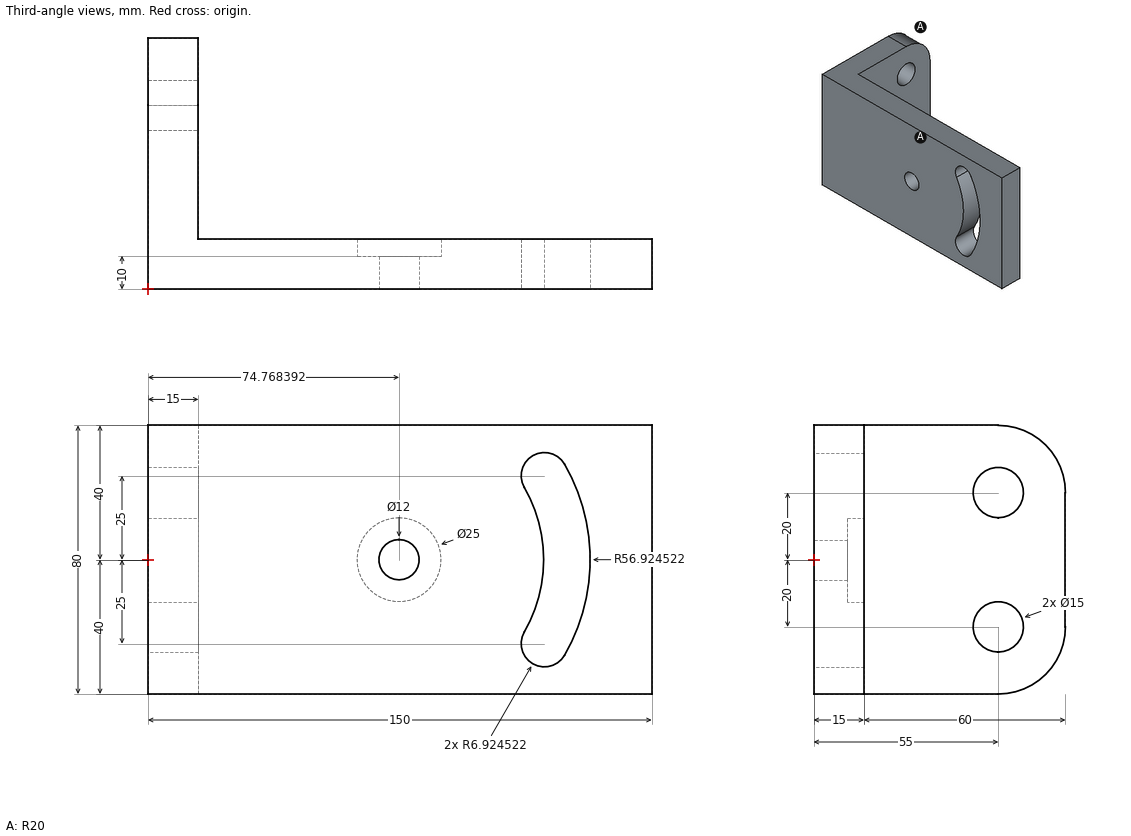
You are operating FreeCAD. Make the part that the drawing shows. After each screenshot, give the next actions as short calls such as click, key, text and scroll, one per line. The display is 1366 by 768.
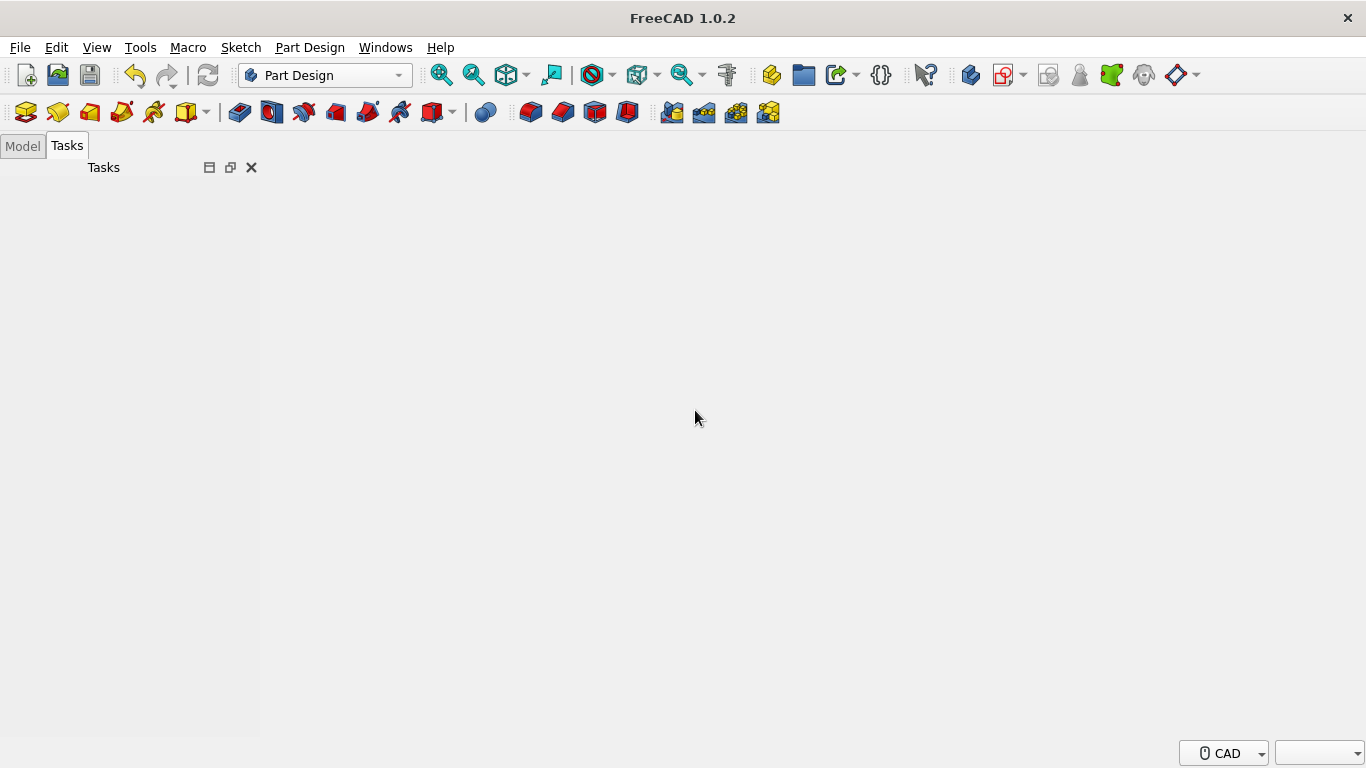
key(ctrl+n)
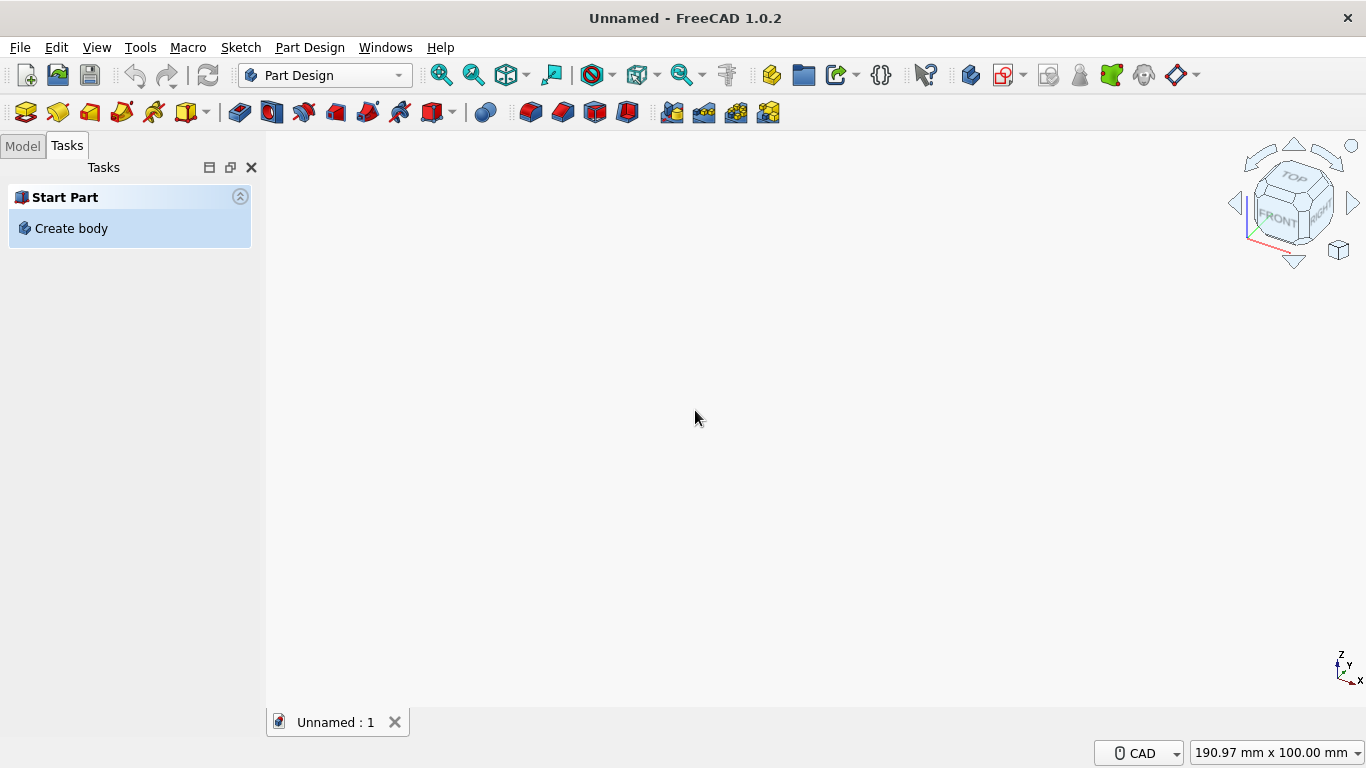
click(1004, 76)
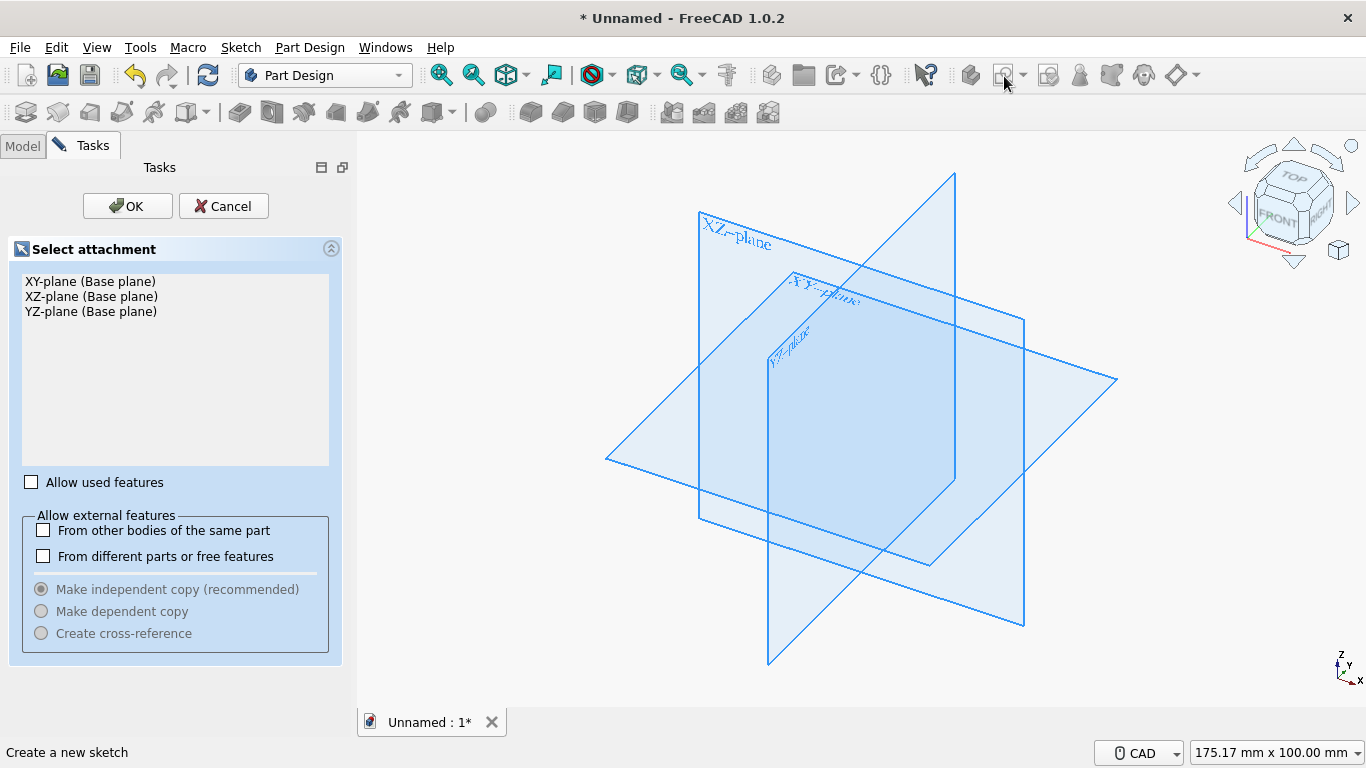
click(82, 296)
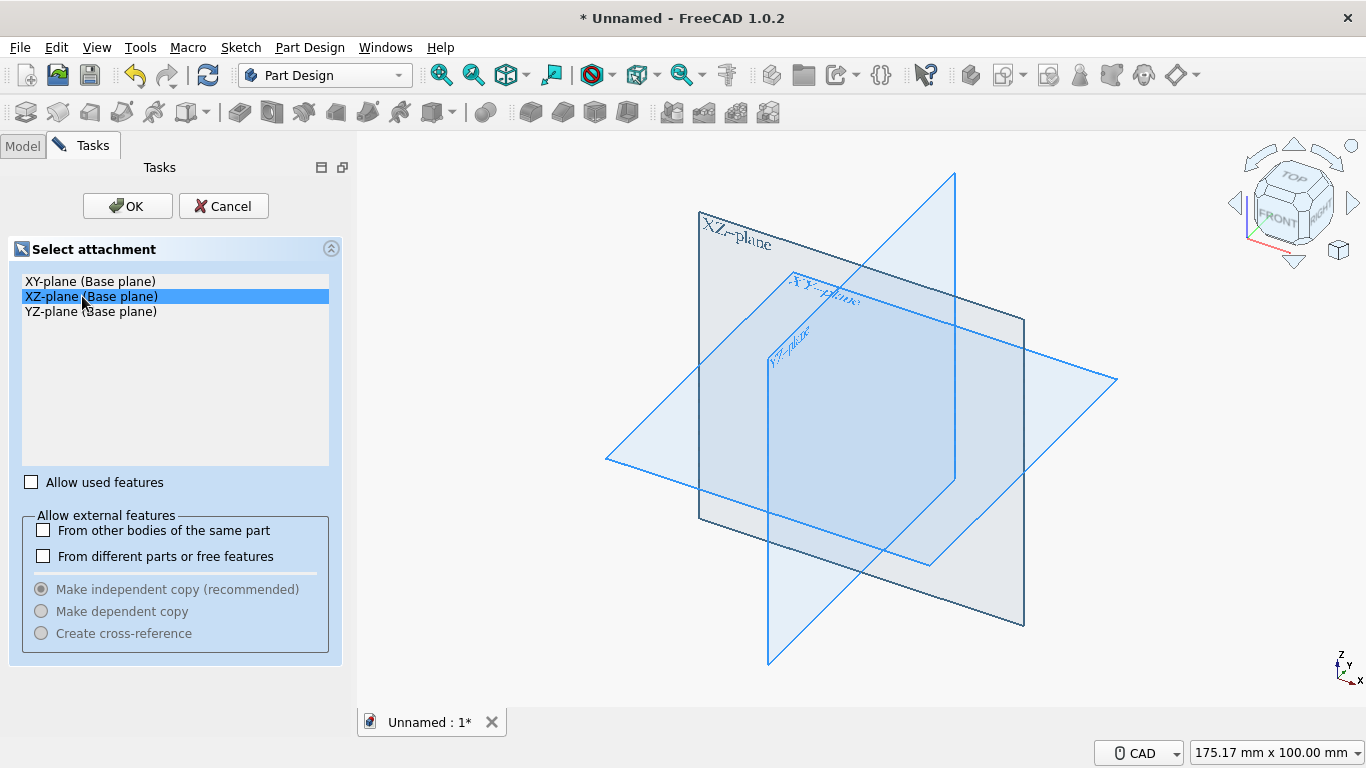
click(128, 206)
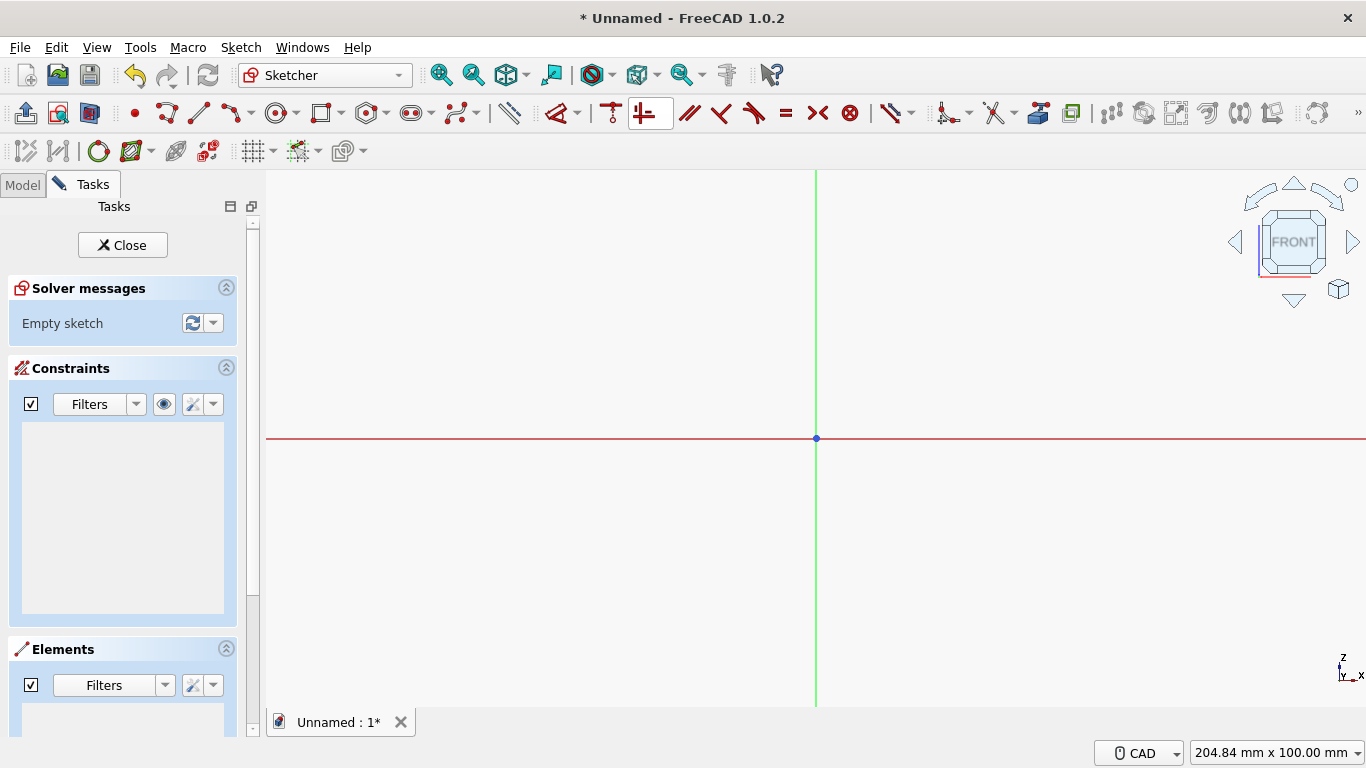
scroll(294, 438, down, 3)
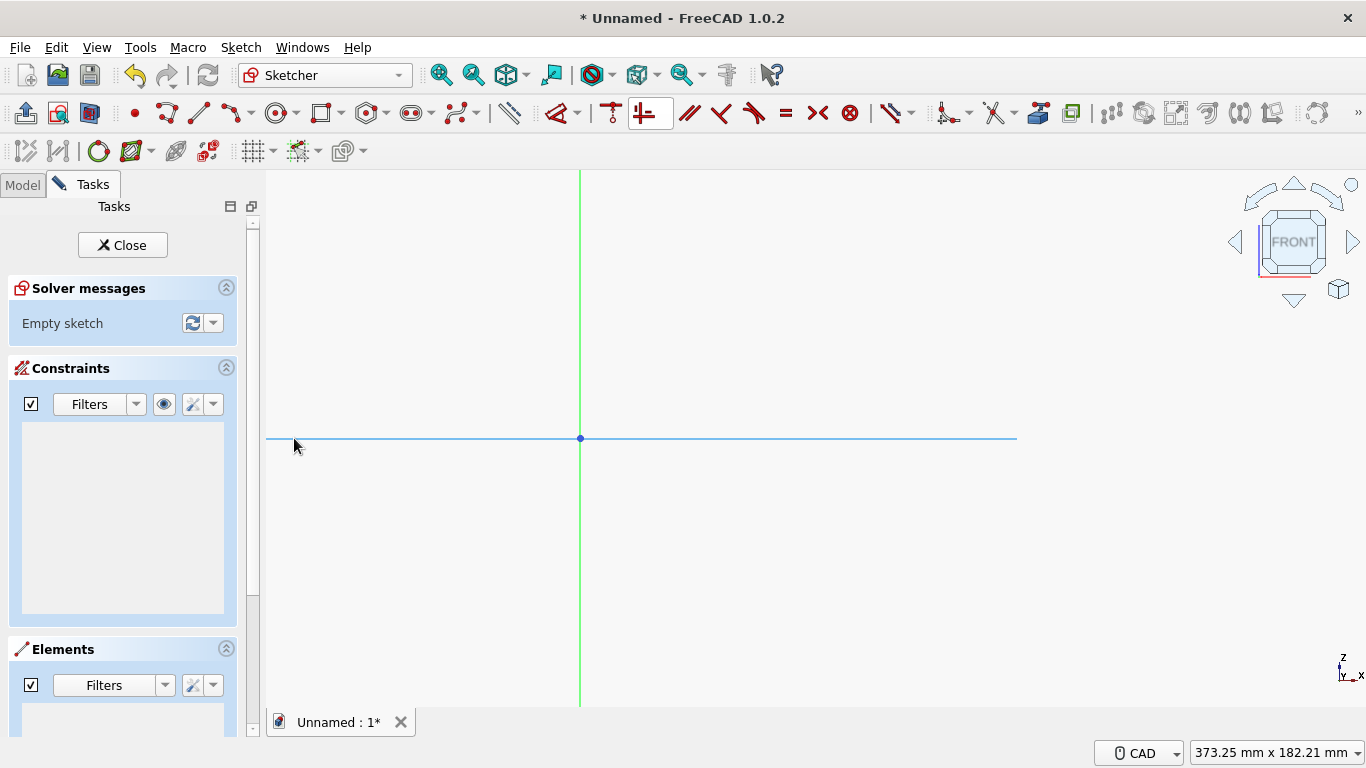
scroll(911, 439, up, 2)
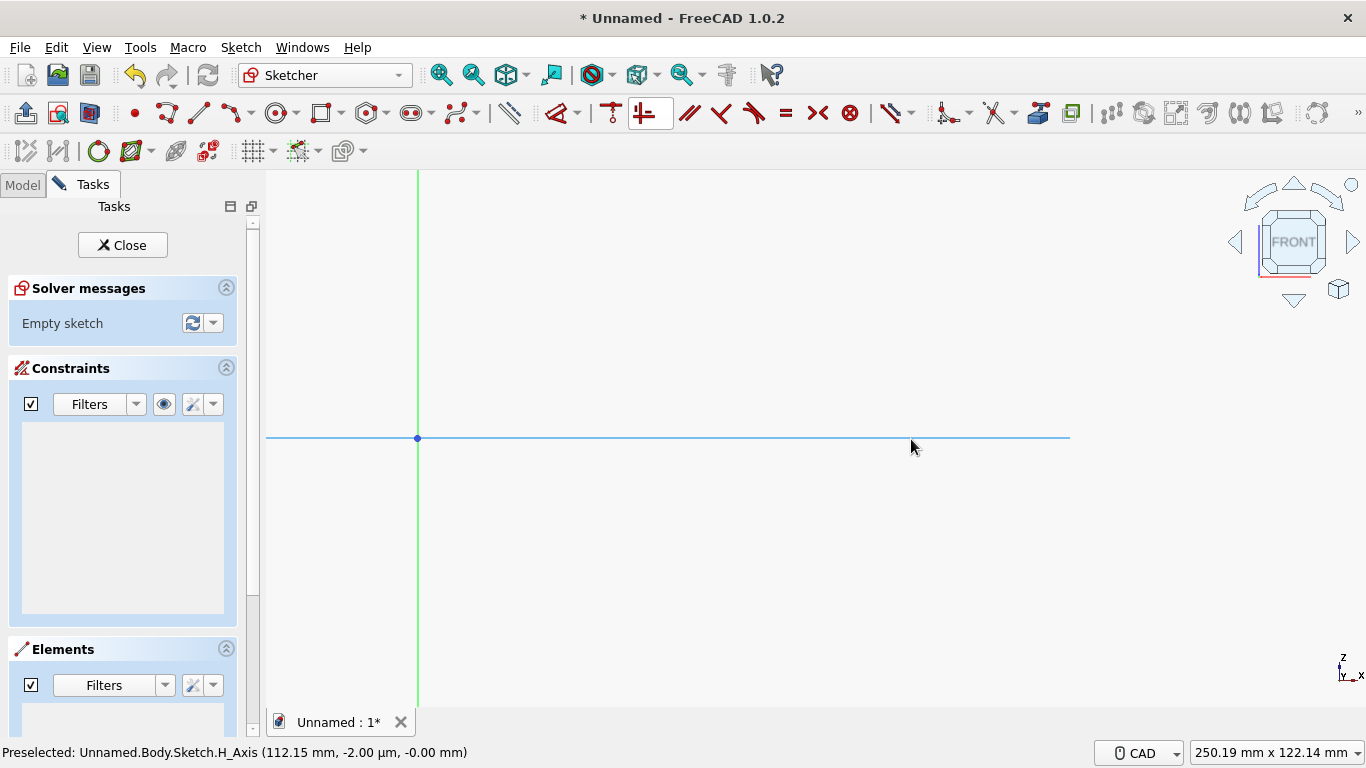
click(322, 114)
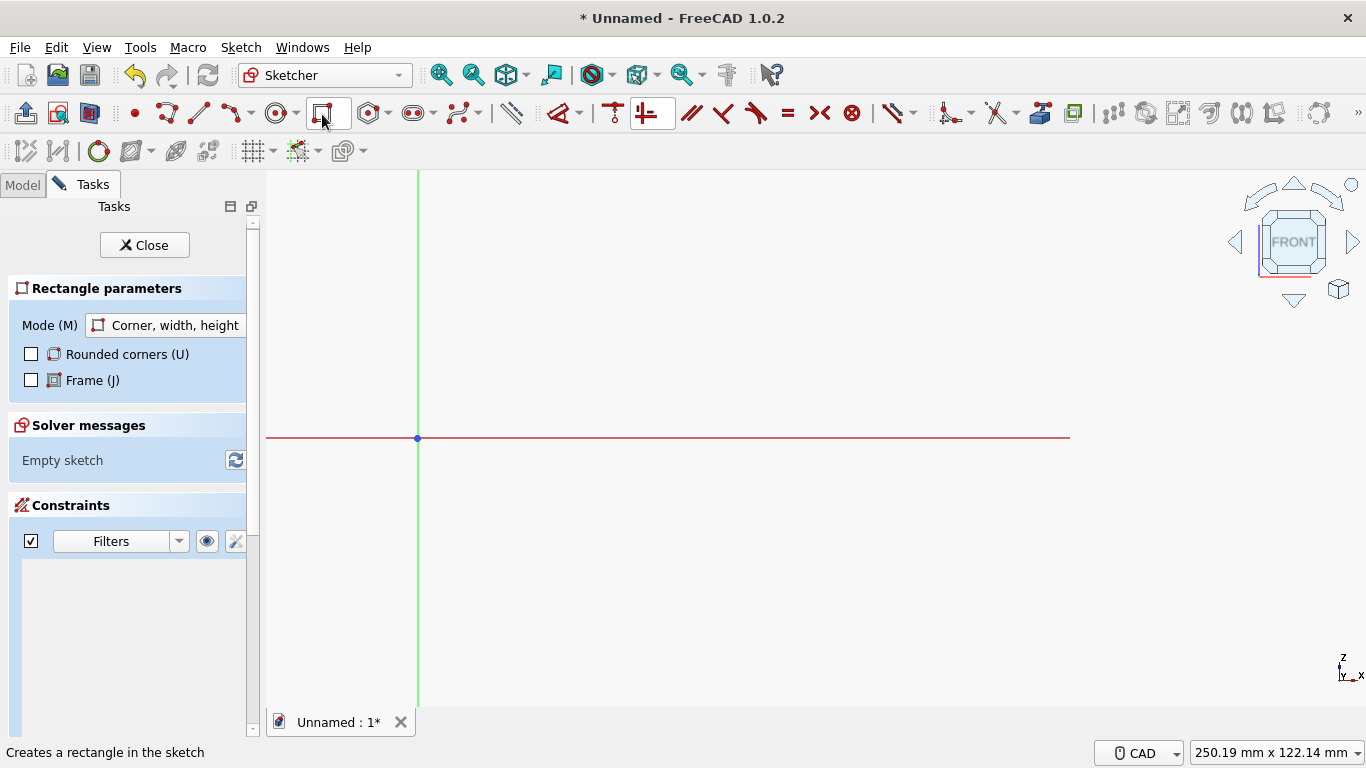
click(418, 262)
click(1077, 614)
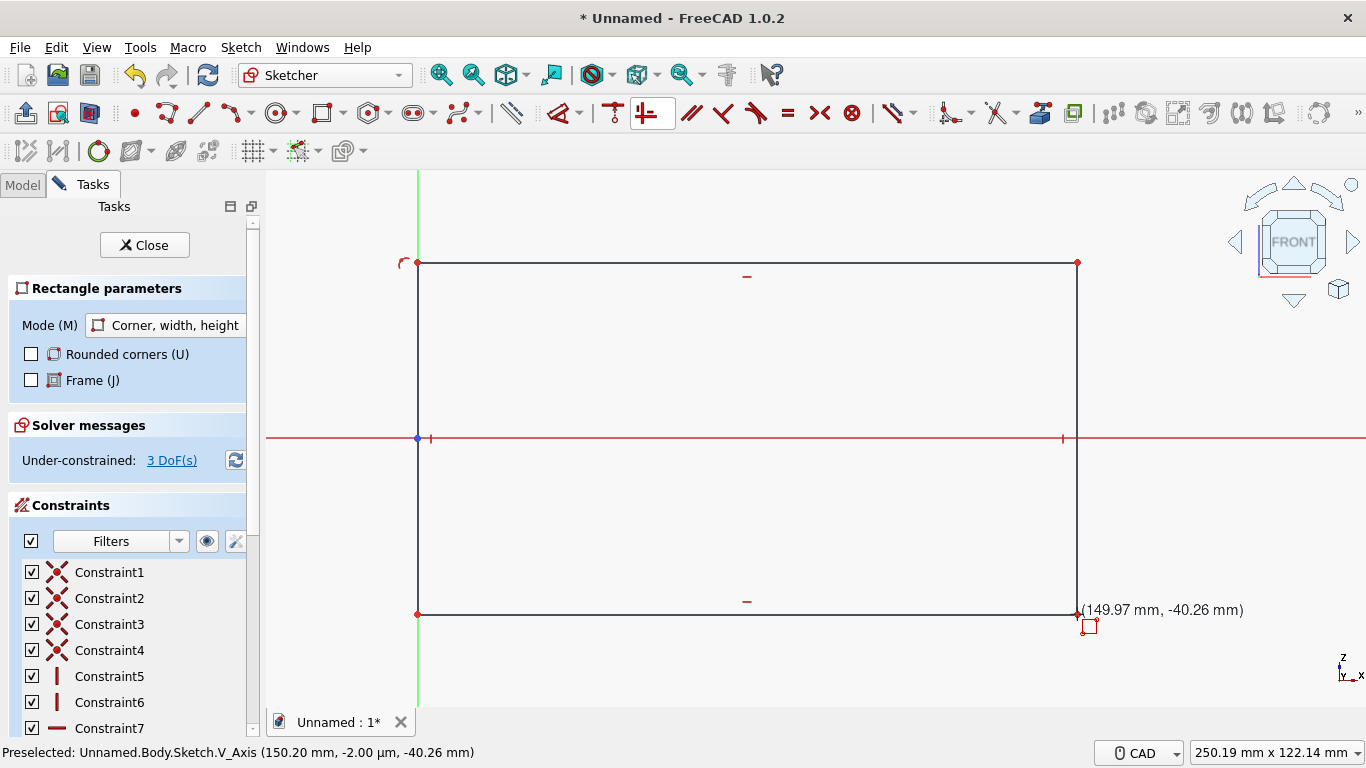
click(232, 114)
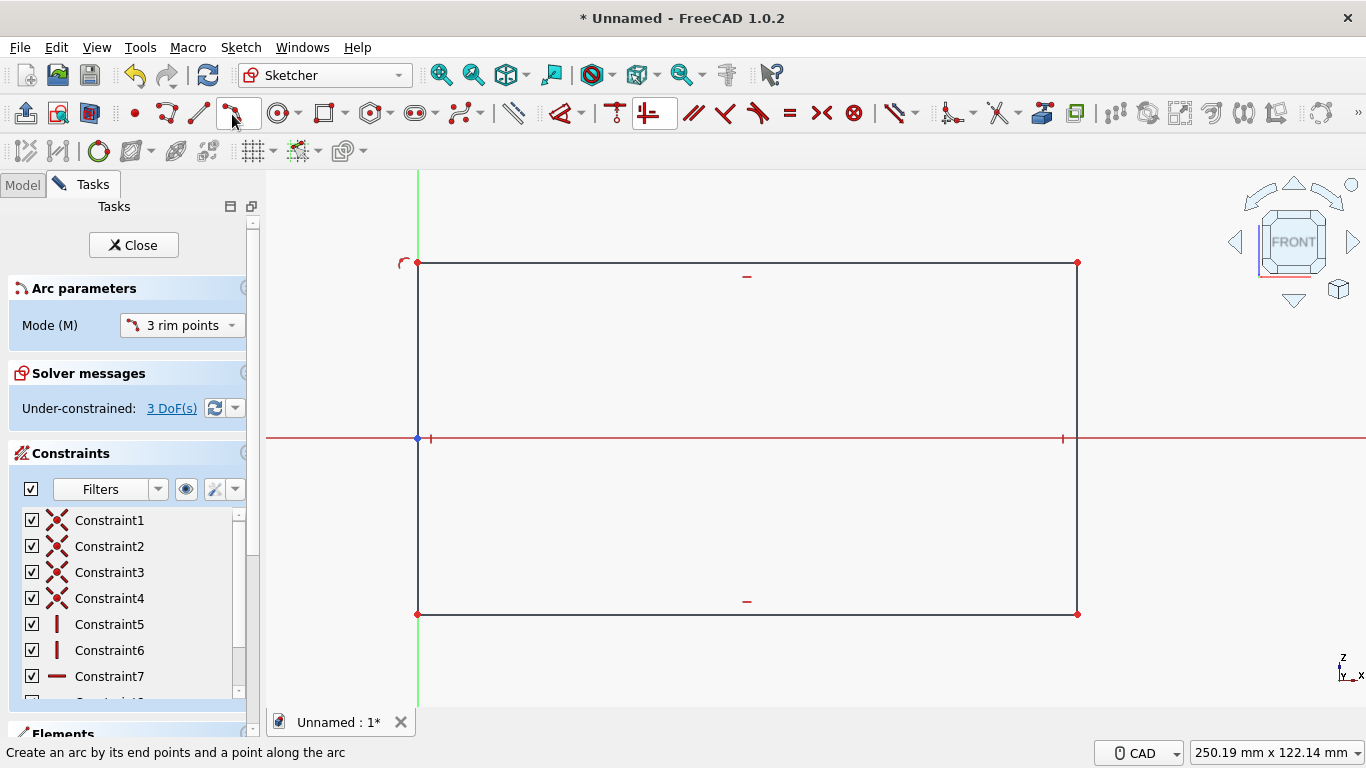
click(910, 533)
click(963, 563)
click(922, 574)